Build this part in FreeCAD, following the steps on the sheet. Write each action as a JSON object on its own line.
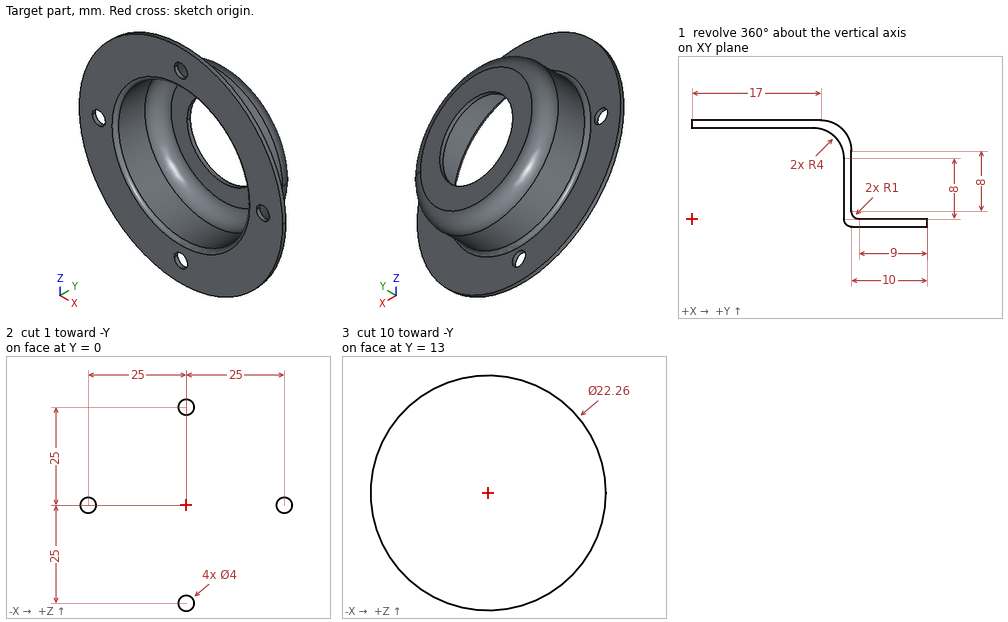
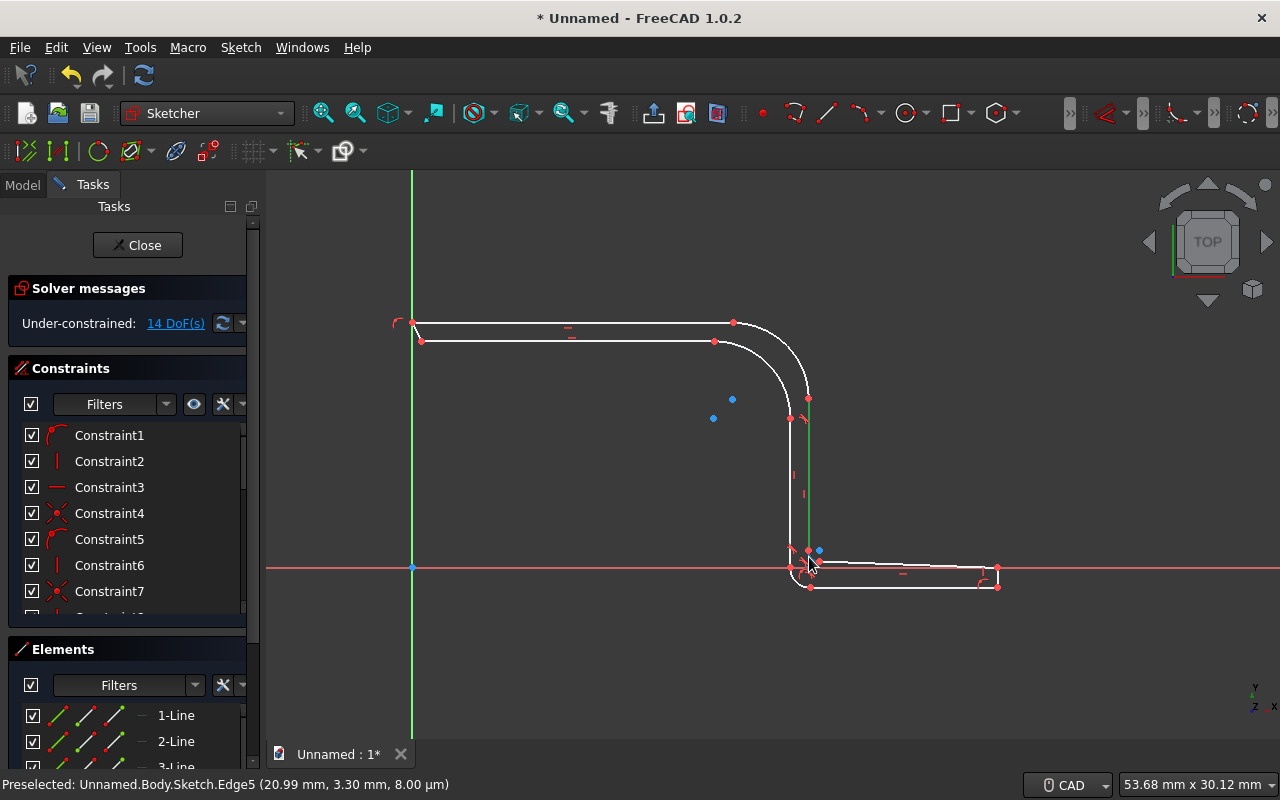
{"action": "left_click", "coordinate": [800, 365]}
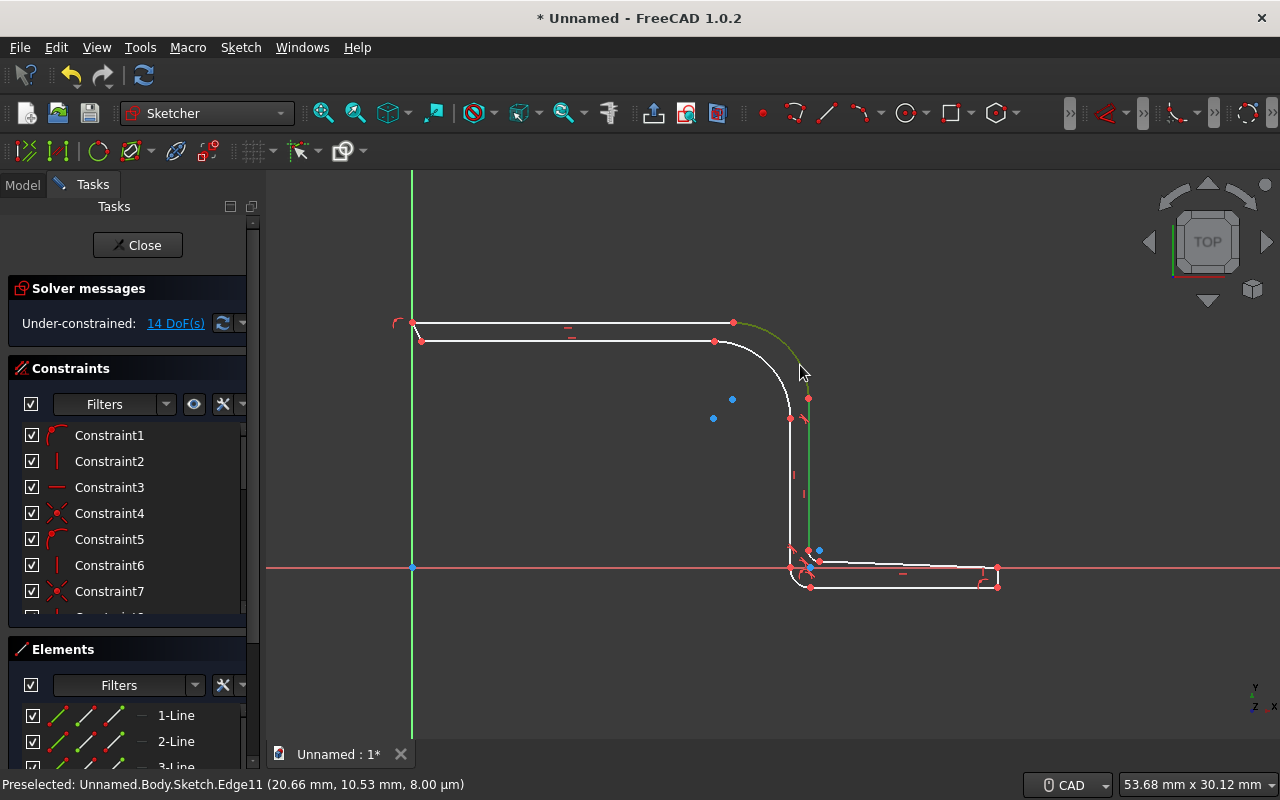
{"action": "key", "text": "t"}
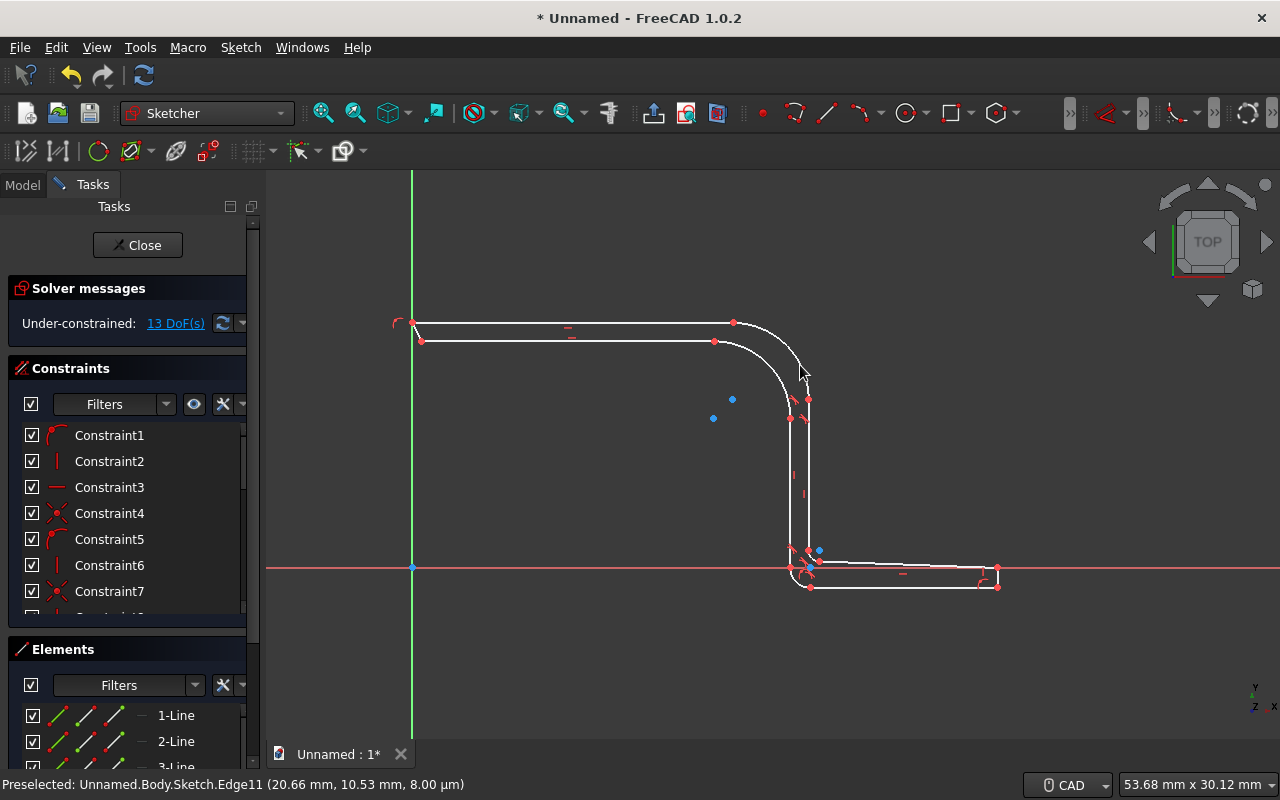
{"action": "left_click", "coordinate": [637, 323]}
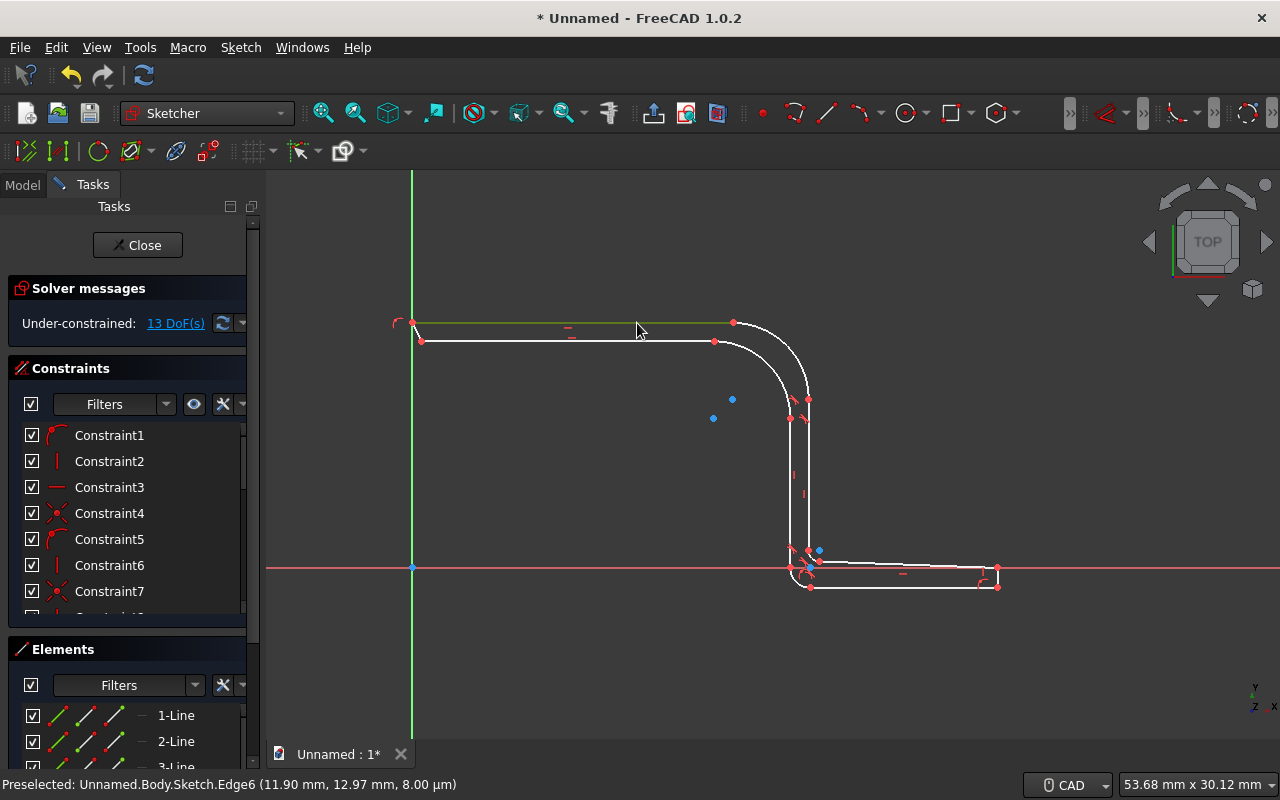
{"action": "left_click", "coordinate": [801, 365]}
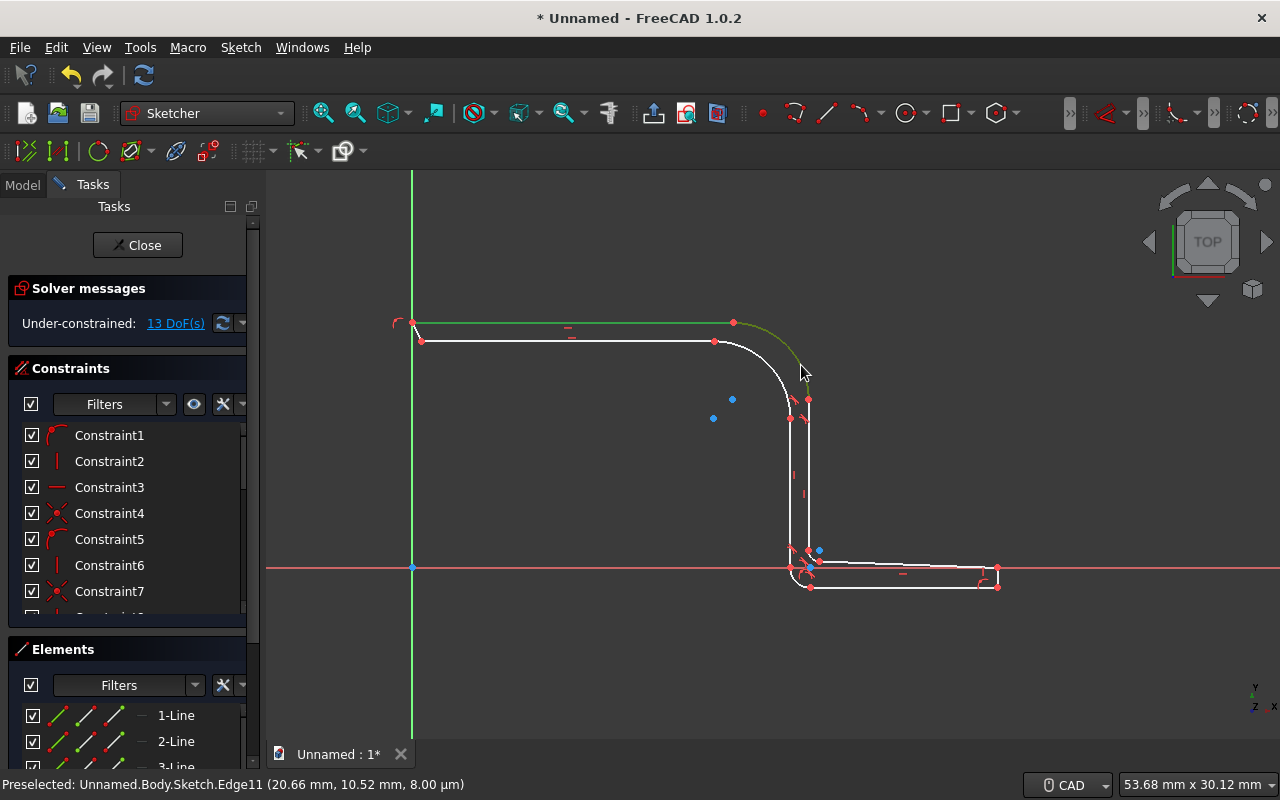
{"action": "key", "text": "t"}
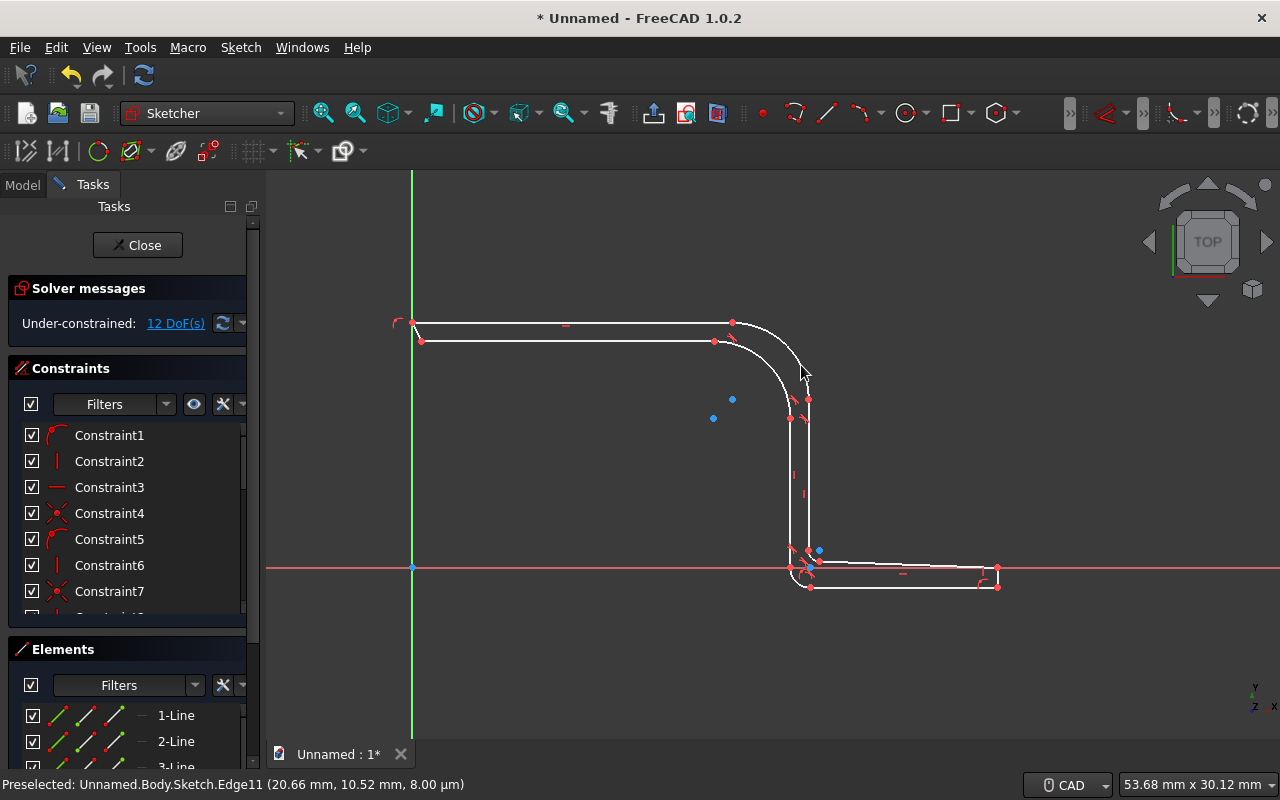
{"action": "left_click", "coordinate": [510, 341]}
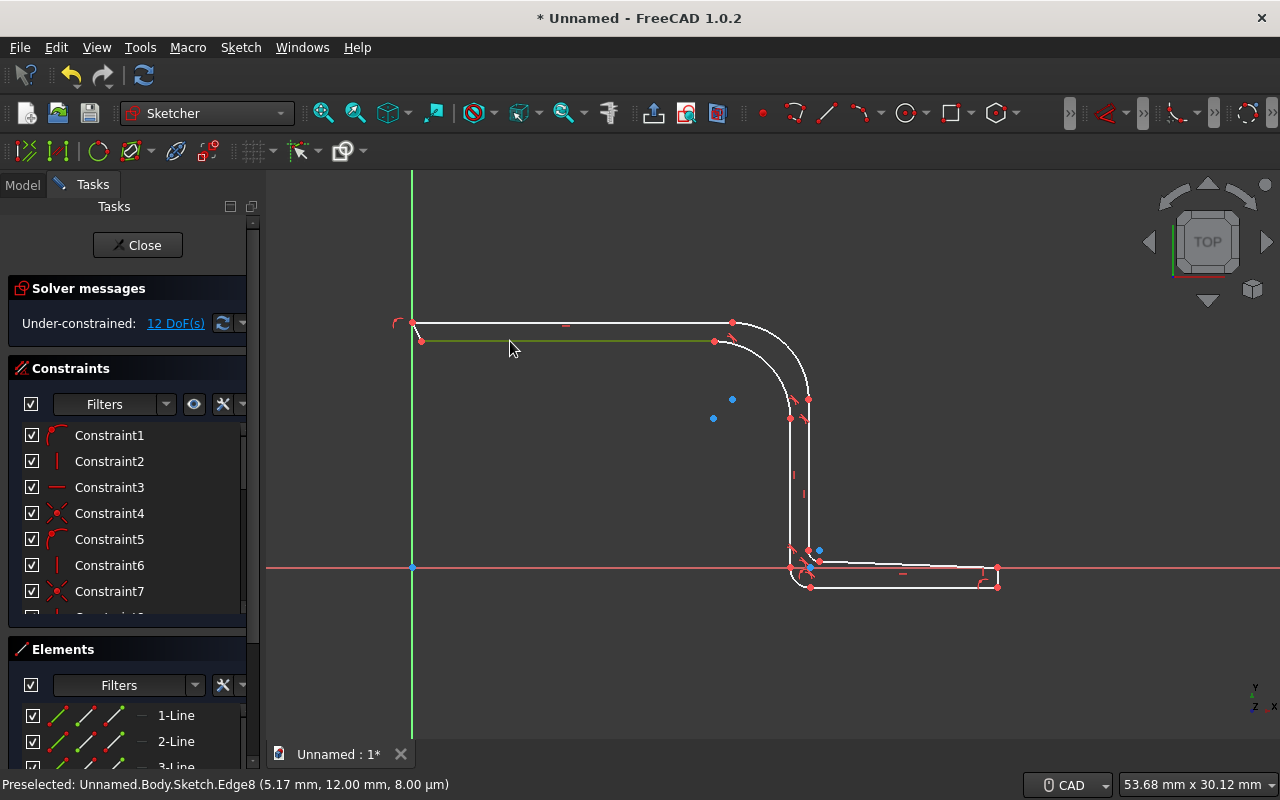
{"action": "left_click", "coordinate": [782, 384]}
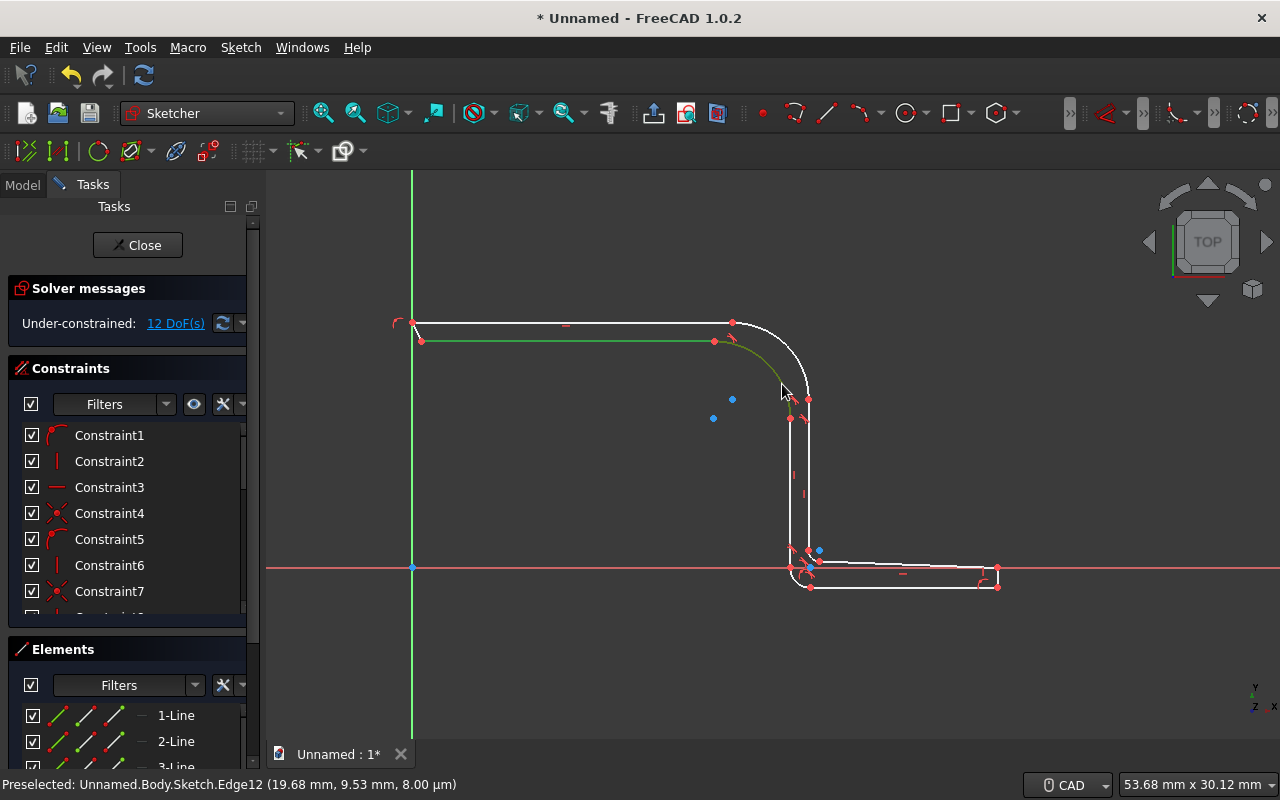
{"action": "key", "text": "t"}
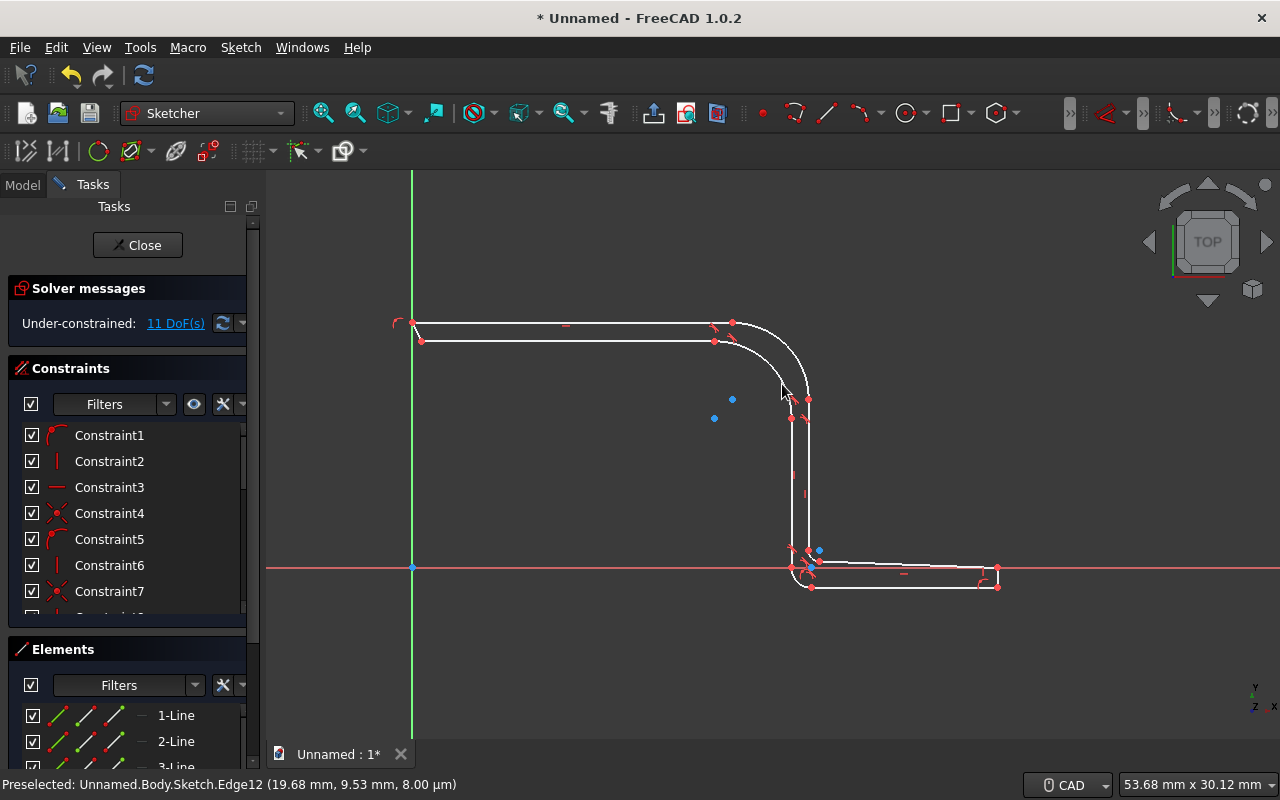
{"action": "left_click", "coordinate": [944, 566]}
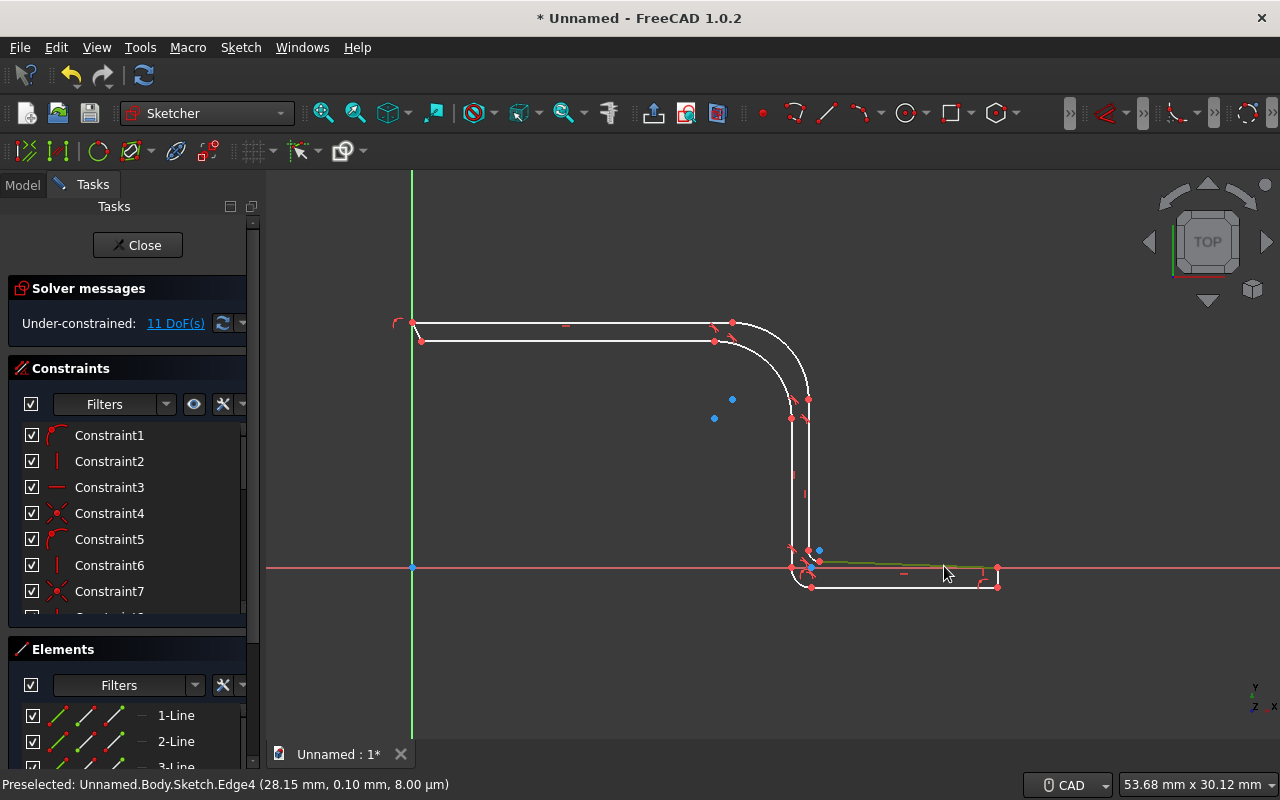
{"action": "key", "text": "h"}